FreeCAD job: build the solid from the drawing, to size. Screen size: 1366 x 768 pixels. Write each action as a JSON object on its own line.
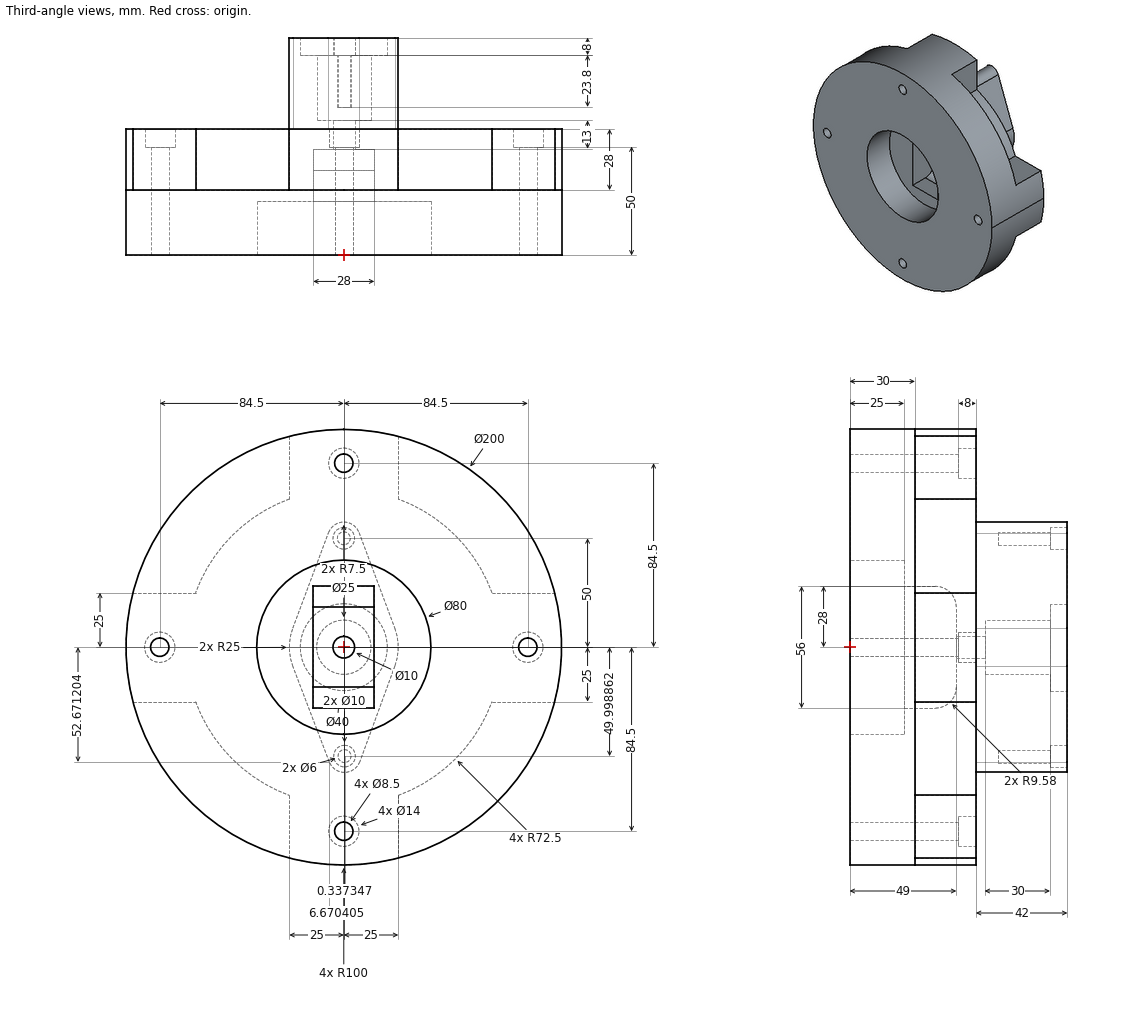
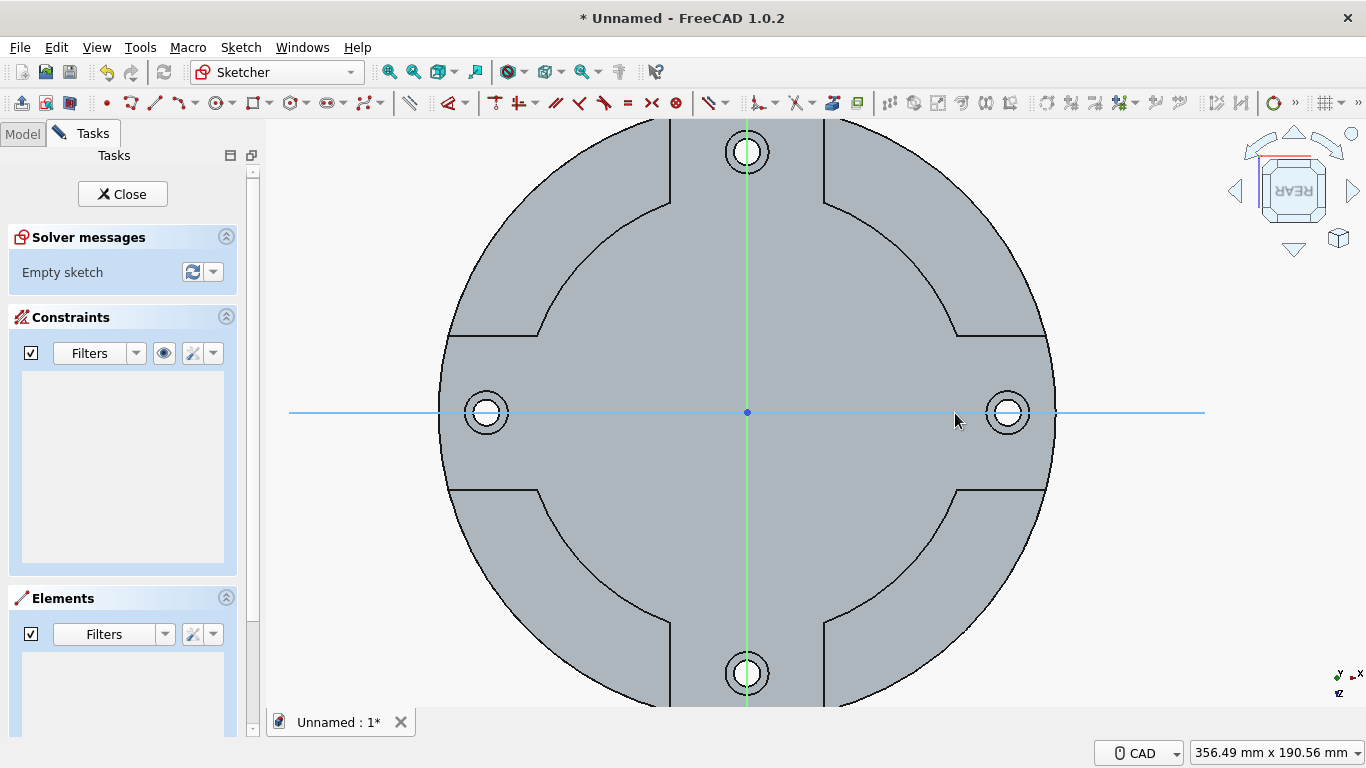
{"action": "key", "text": "g l"}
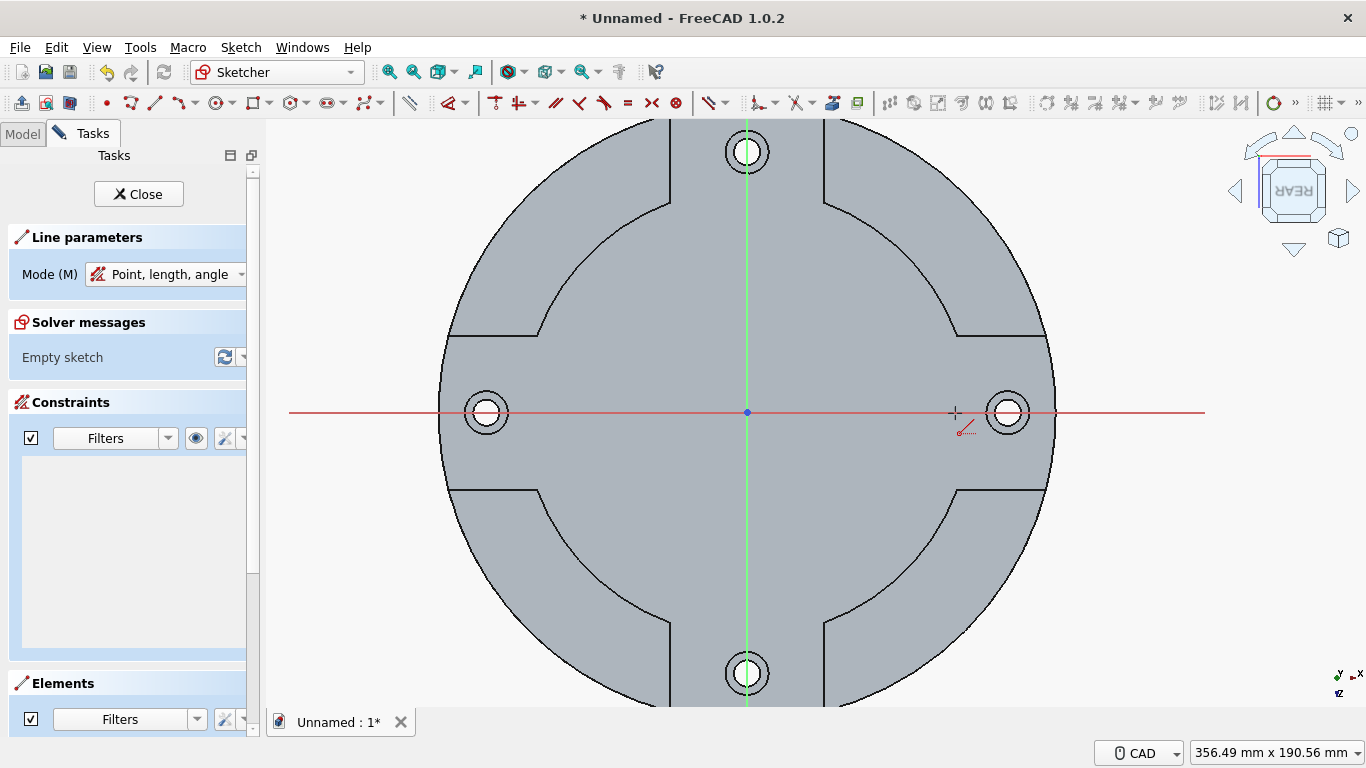
{"action": "left_click", "coordinate": [727, 250]}
{"action": "left_click", "coordinate": [675, 385]}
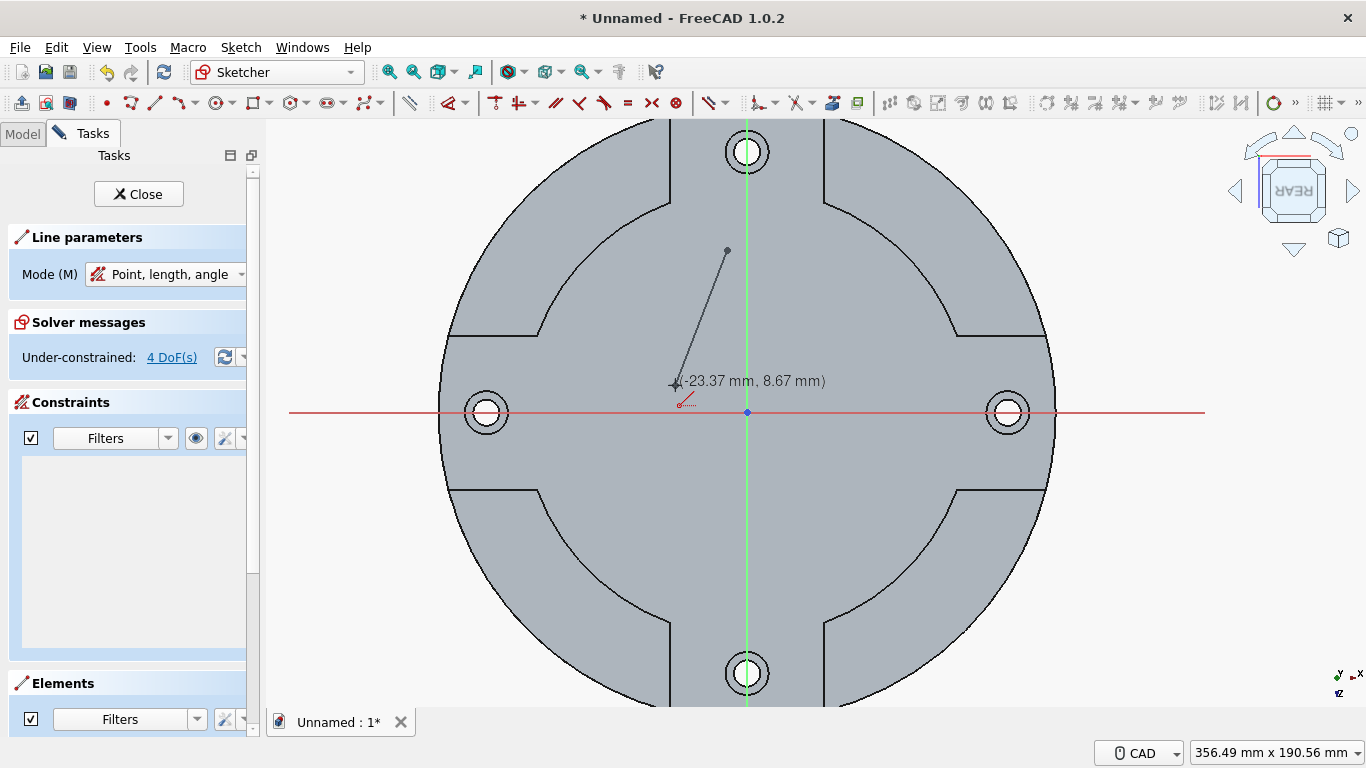
{"action": "left_click", "coordinate": [675, 440]}
{"action": "left_click", "coordinate": [725, 575]}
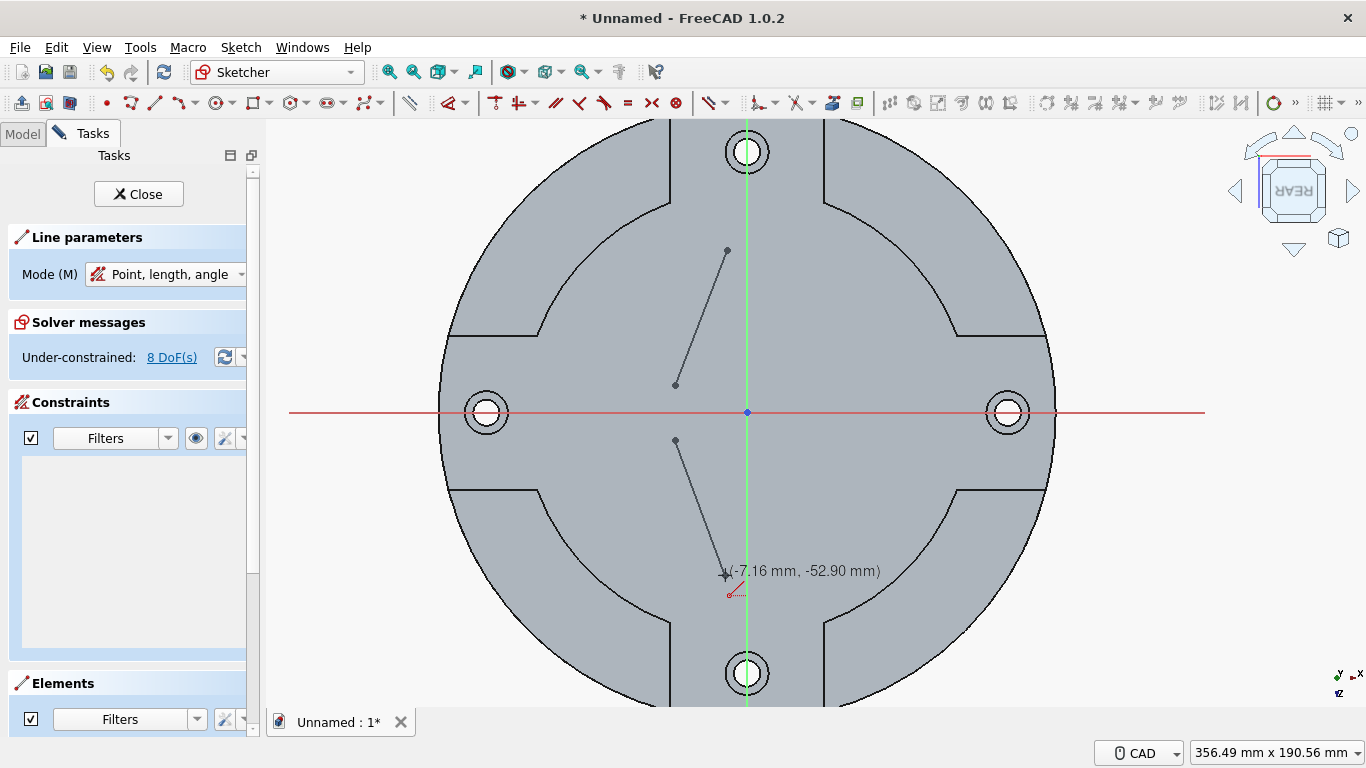
{"action": "left_click", "coordinate": [769, 575]}
{"action": "left_click", "coordinate": [819, 440]}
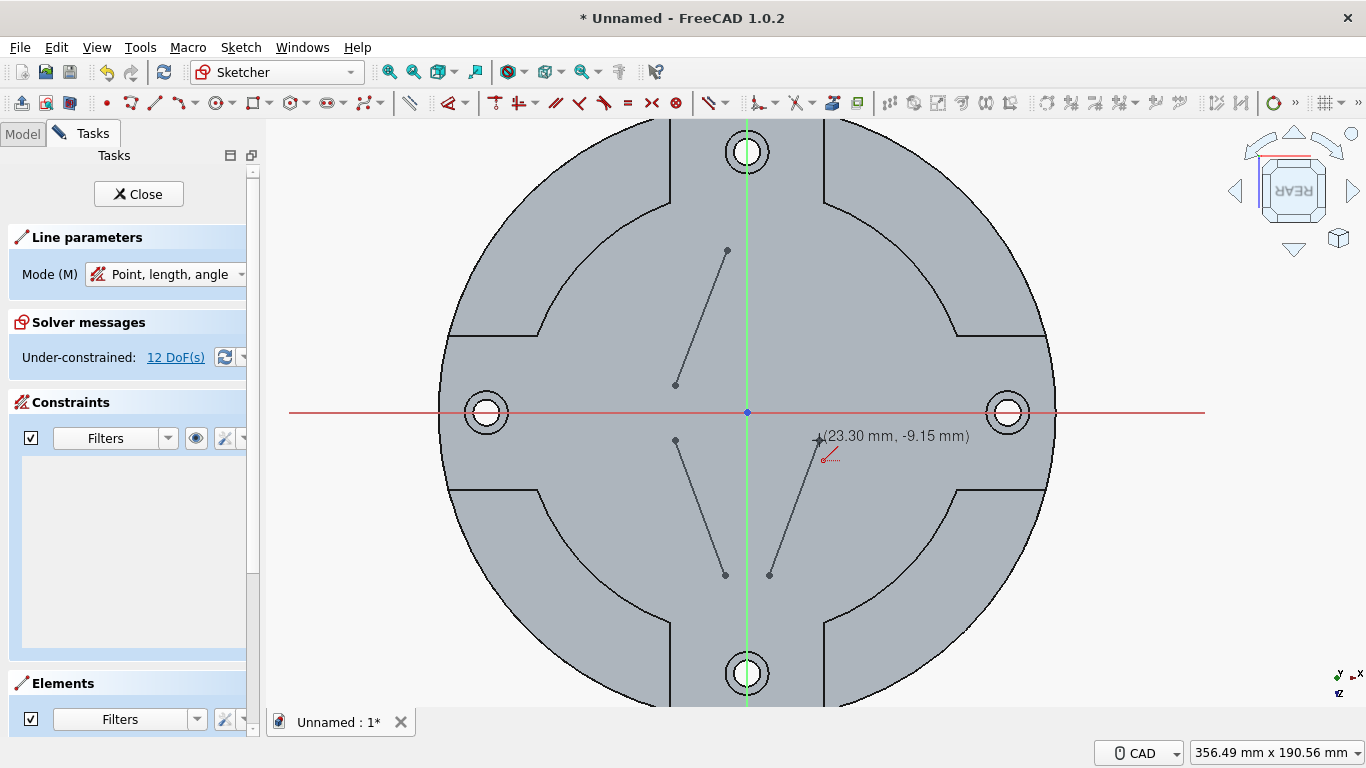
{"action": "left_click", "coordinate": [820, 386]}
{"action": "left_click", "coordinate": [770, 251]}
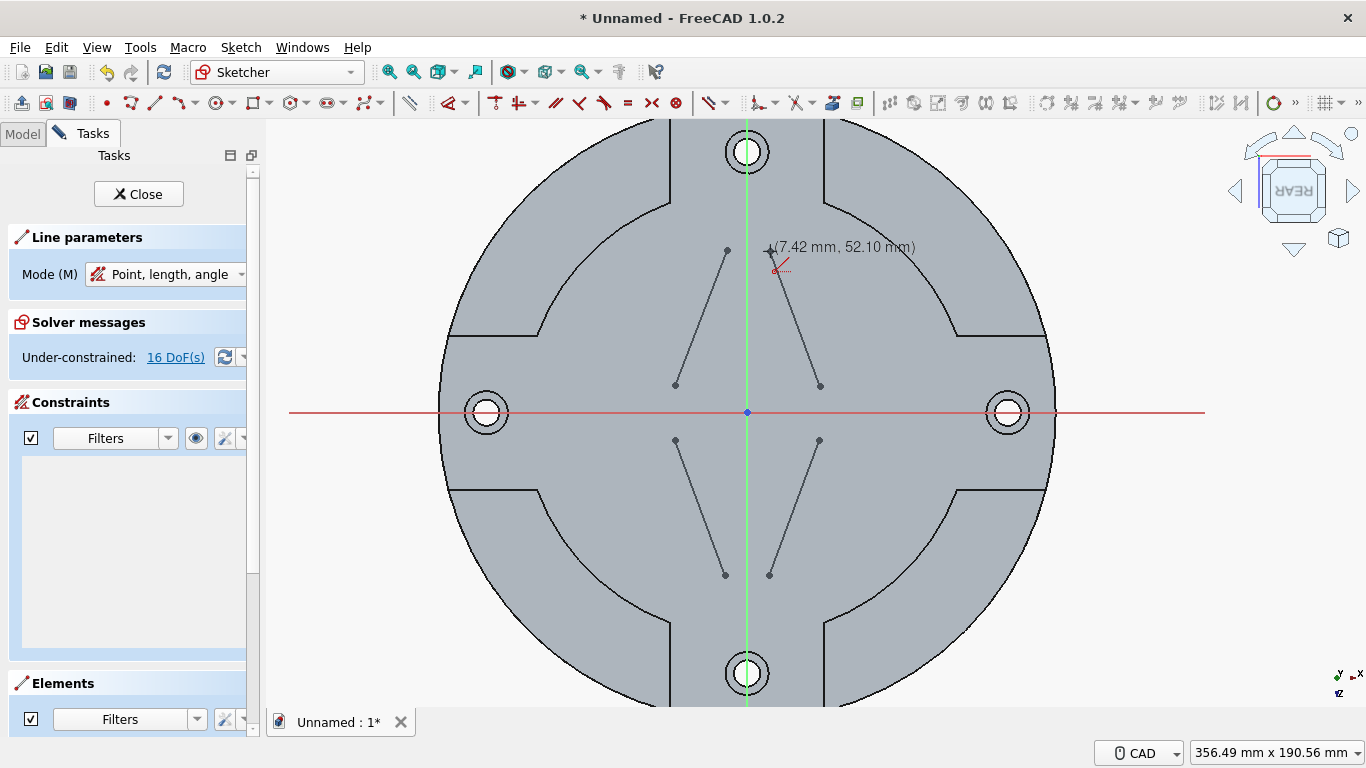
{"action": "key", "text": "g 3 a"}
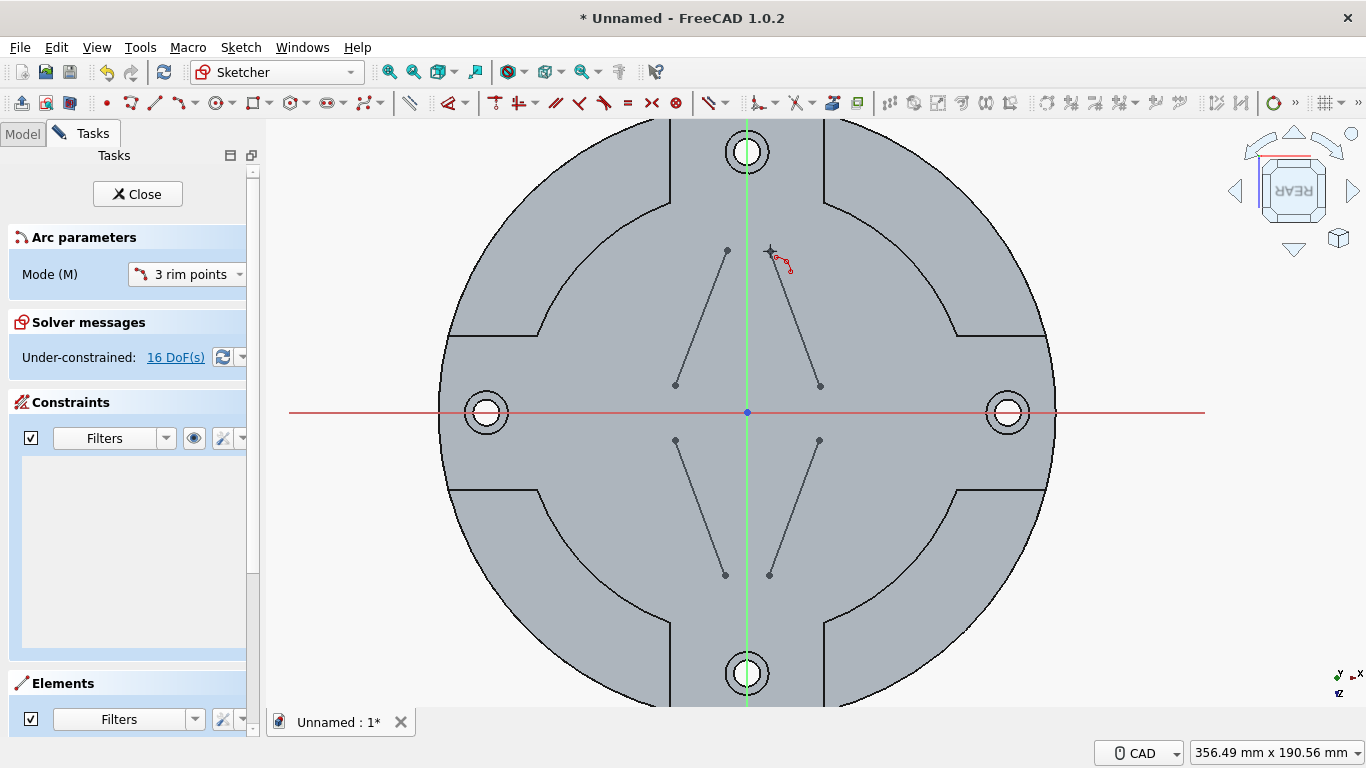
{"action": "left_click", "coordinate": [675, 386]}
{"action": "left_click", "coordinate": [675, 441]}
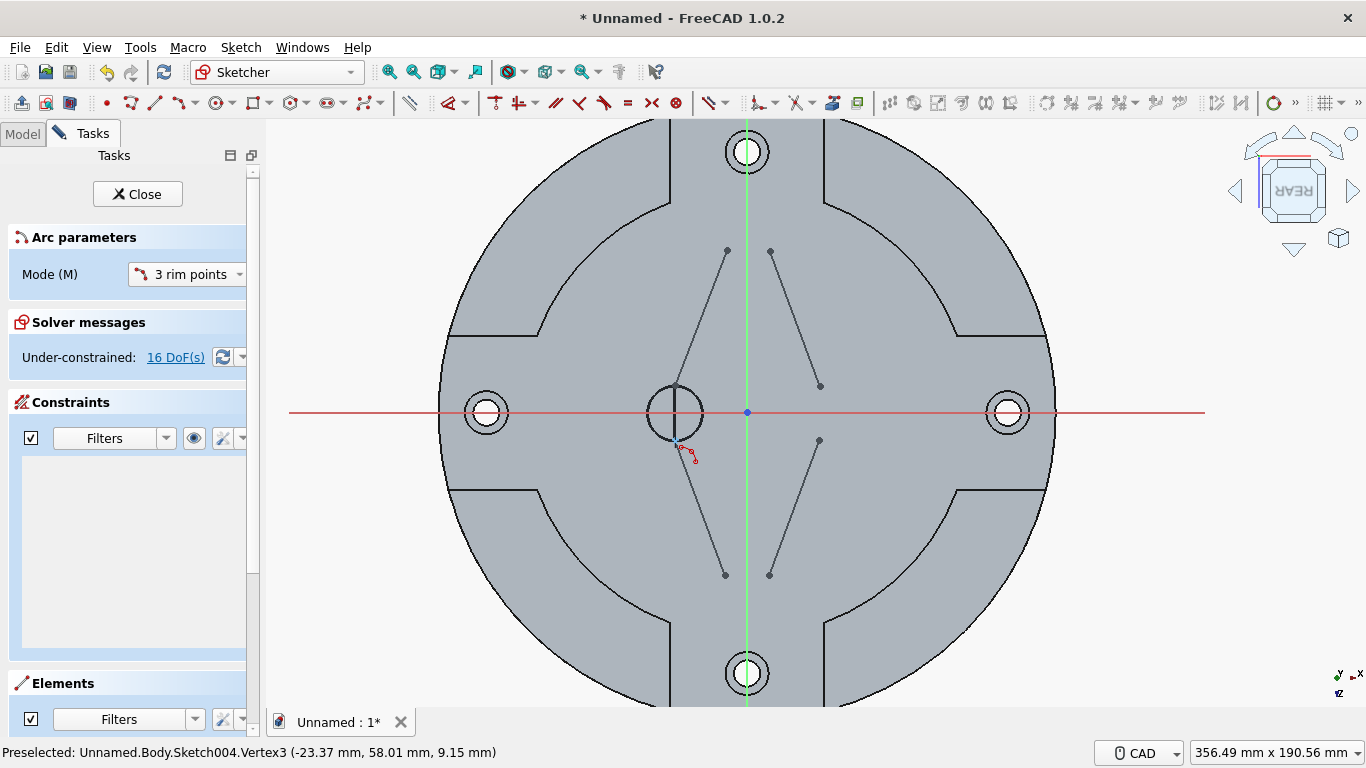
{"action": "scroll", "coordinate": [670, 407], "scroll_direction": "up", "scroll_amount": 7}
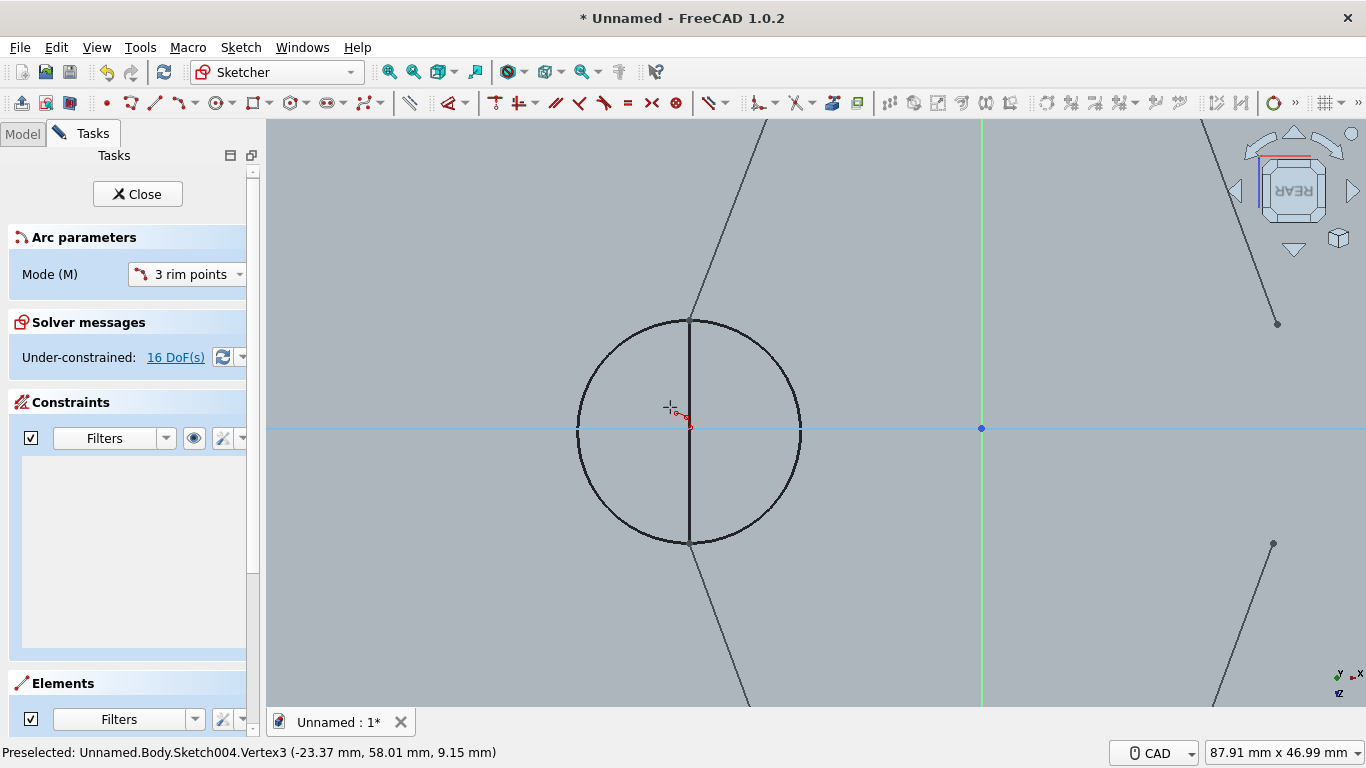
{"action": "left_click", "coordinate": [670, 405]}